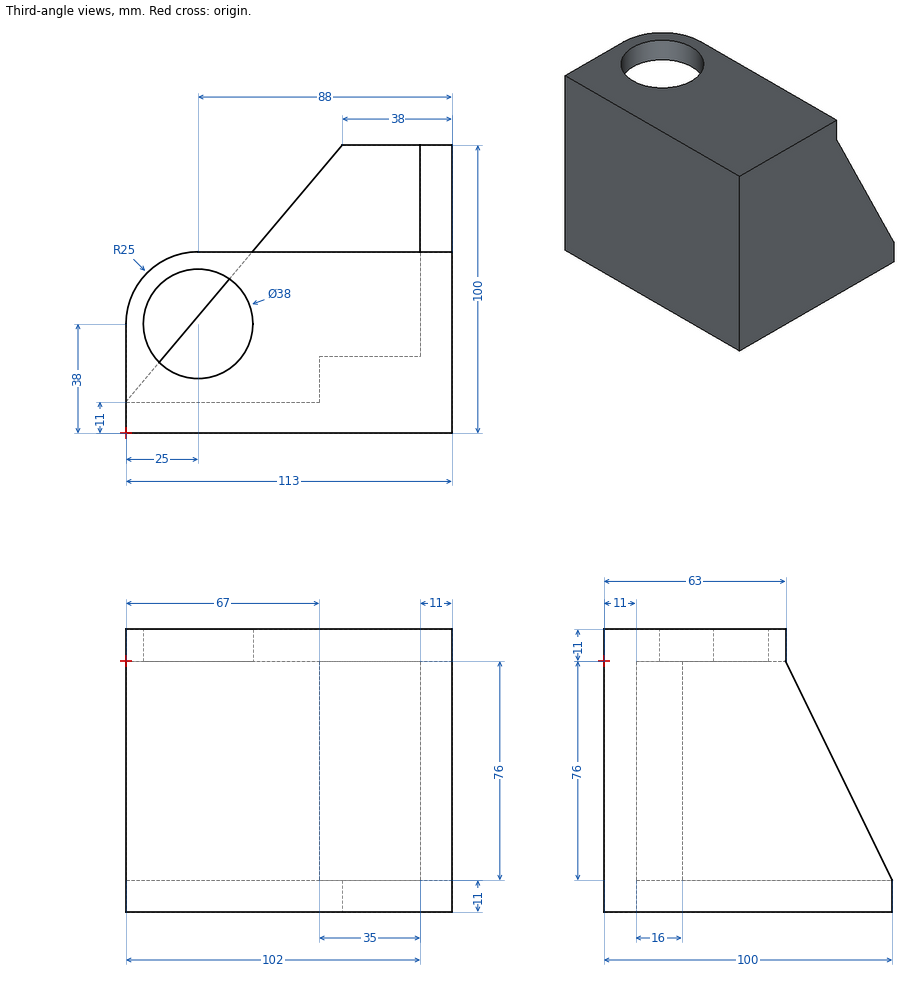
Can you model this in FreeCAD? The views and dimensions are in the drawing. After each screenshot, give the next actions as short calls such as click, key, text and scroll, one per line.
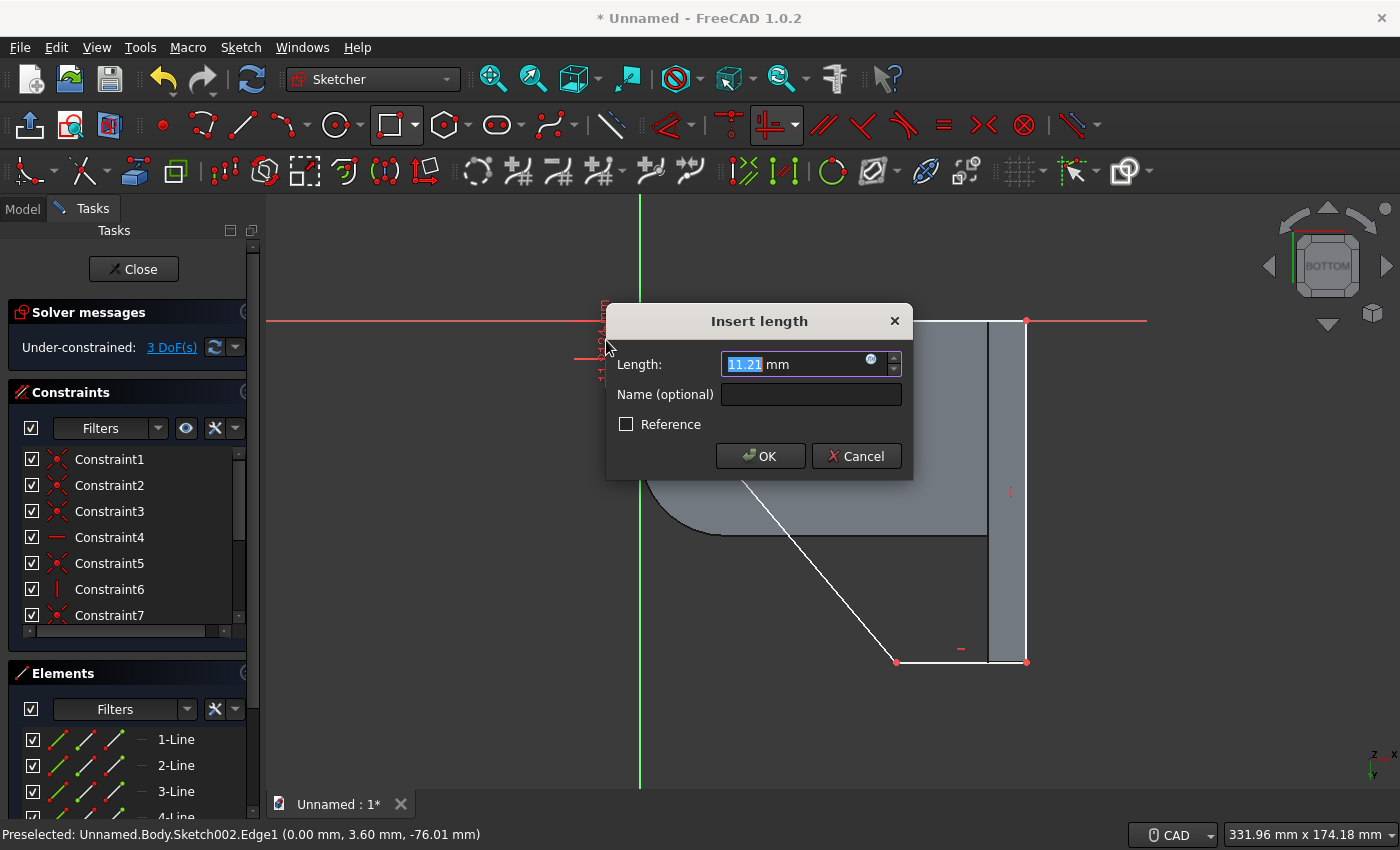
text(11)
key(Return)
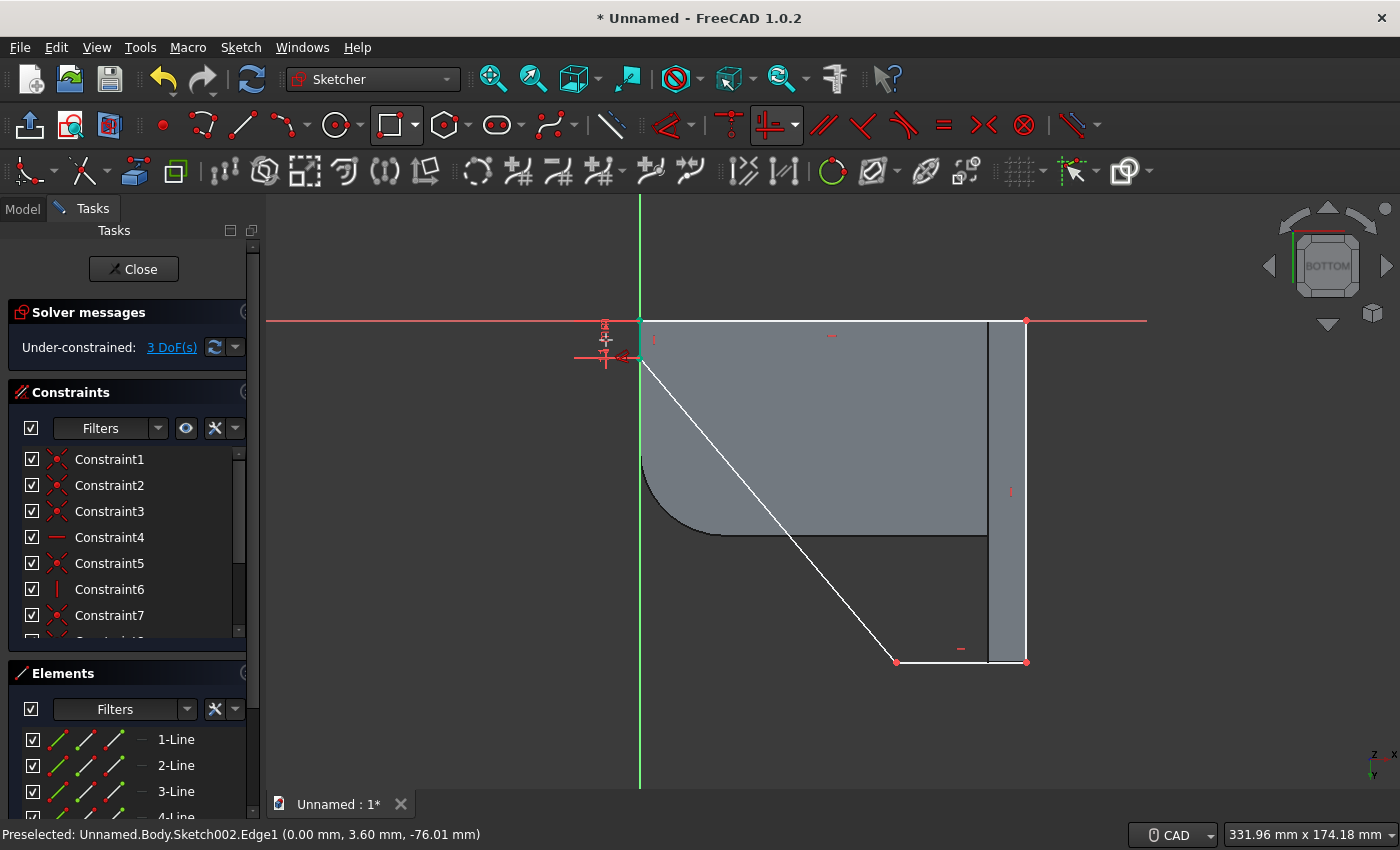
click(935, 663)
click(961, 697)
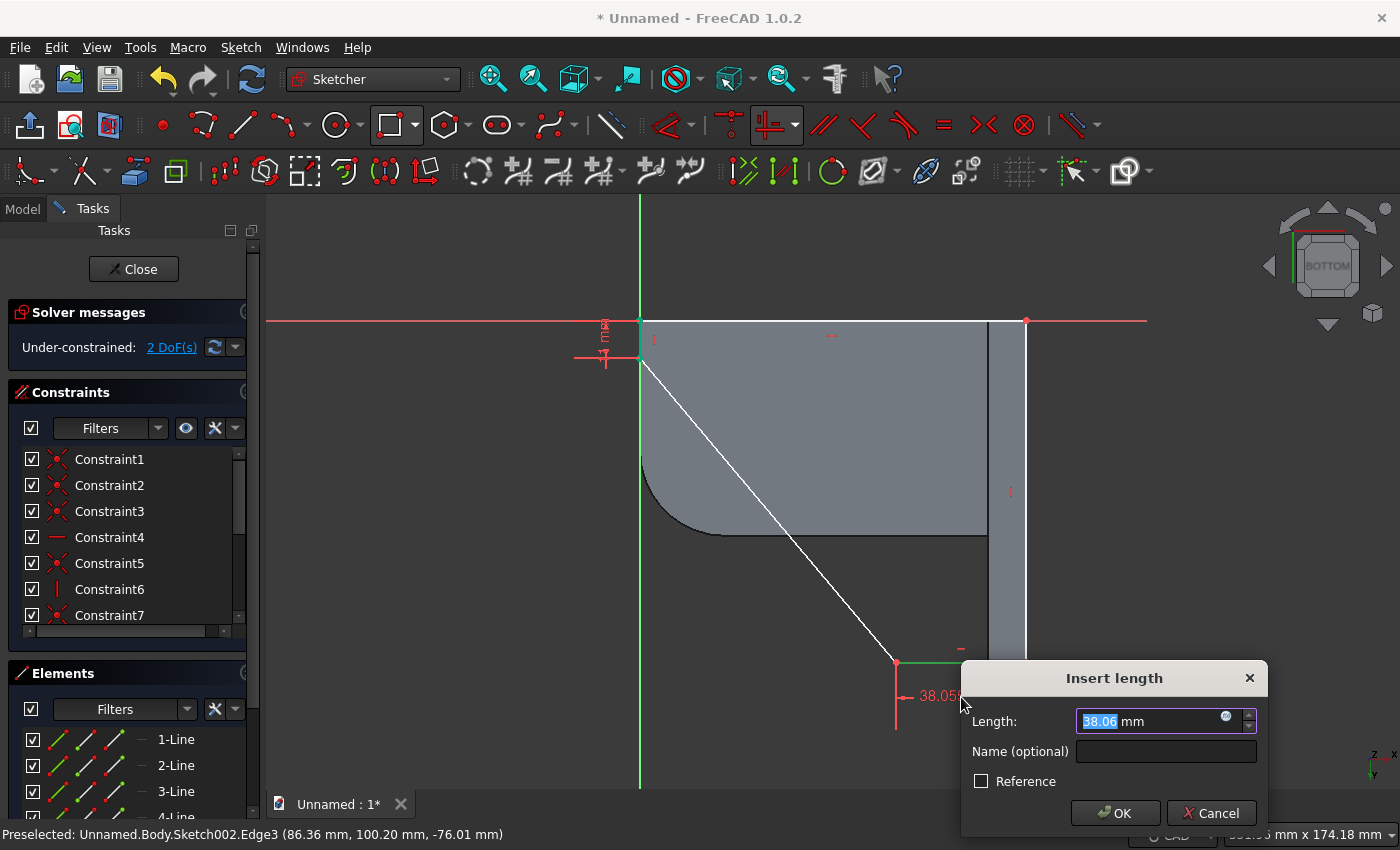
text(38)
key(Return)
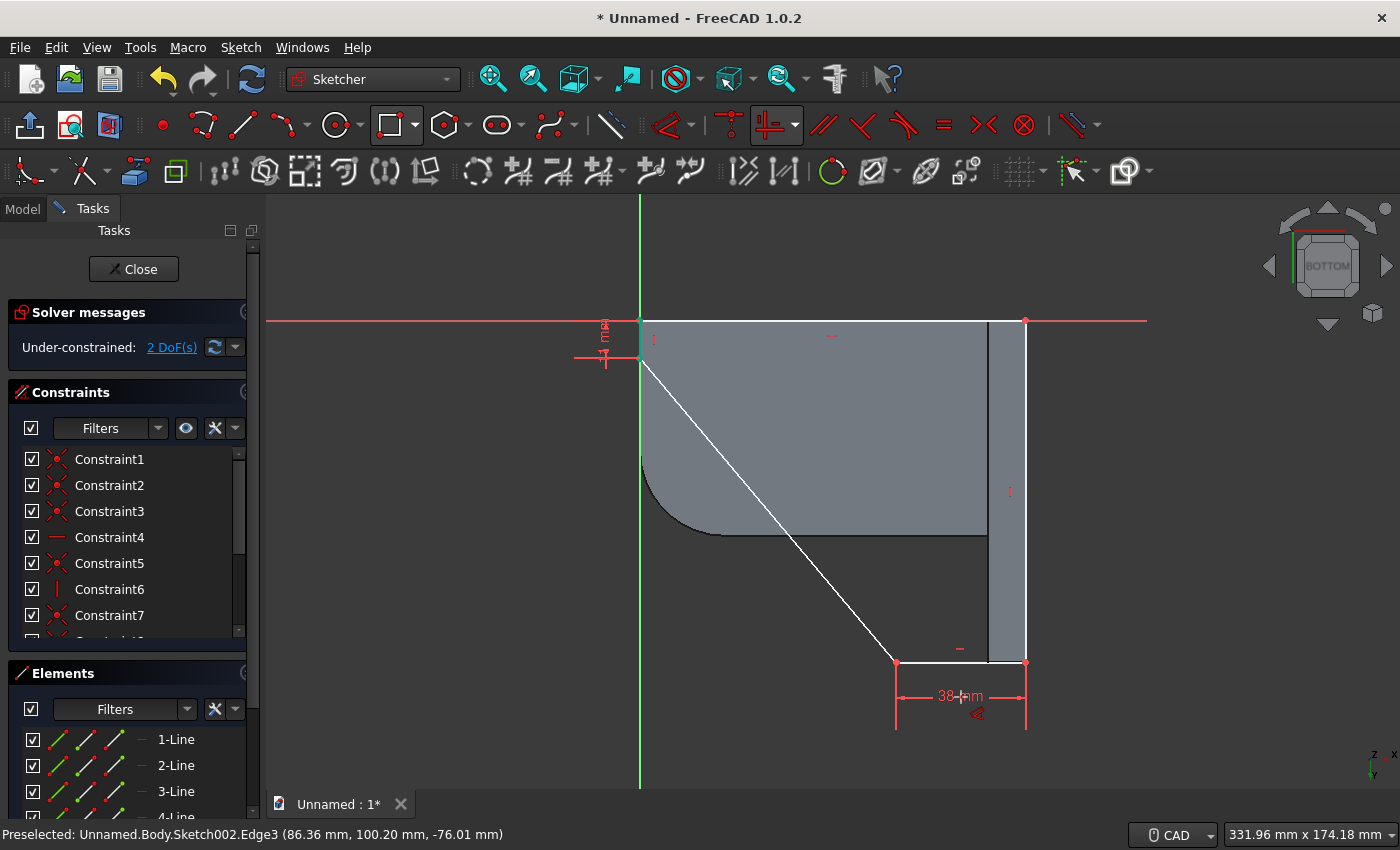
click(1026, 560)
click(1060, 492)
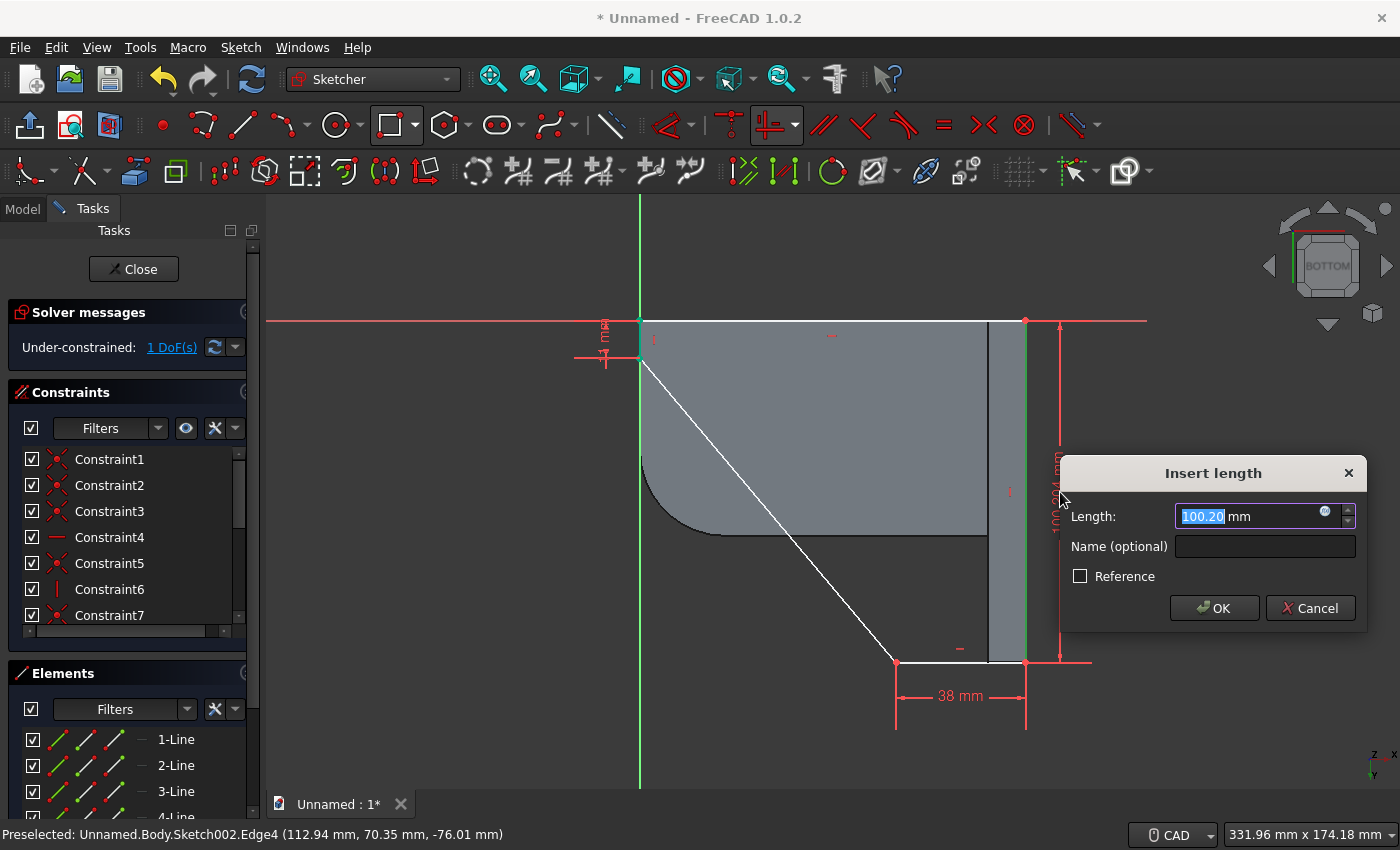
text(100)
key(Return)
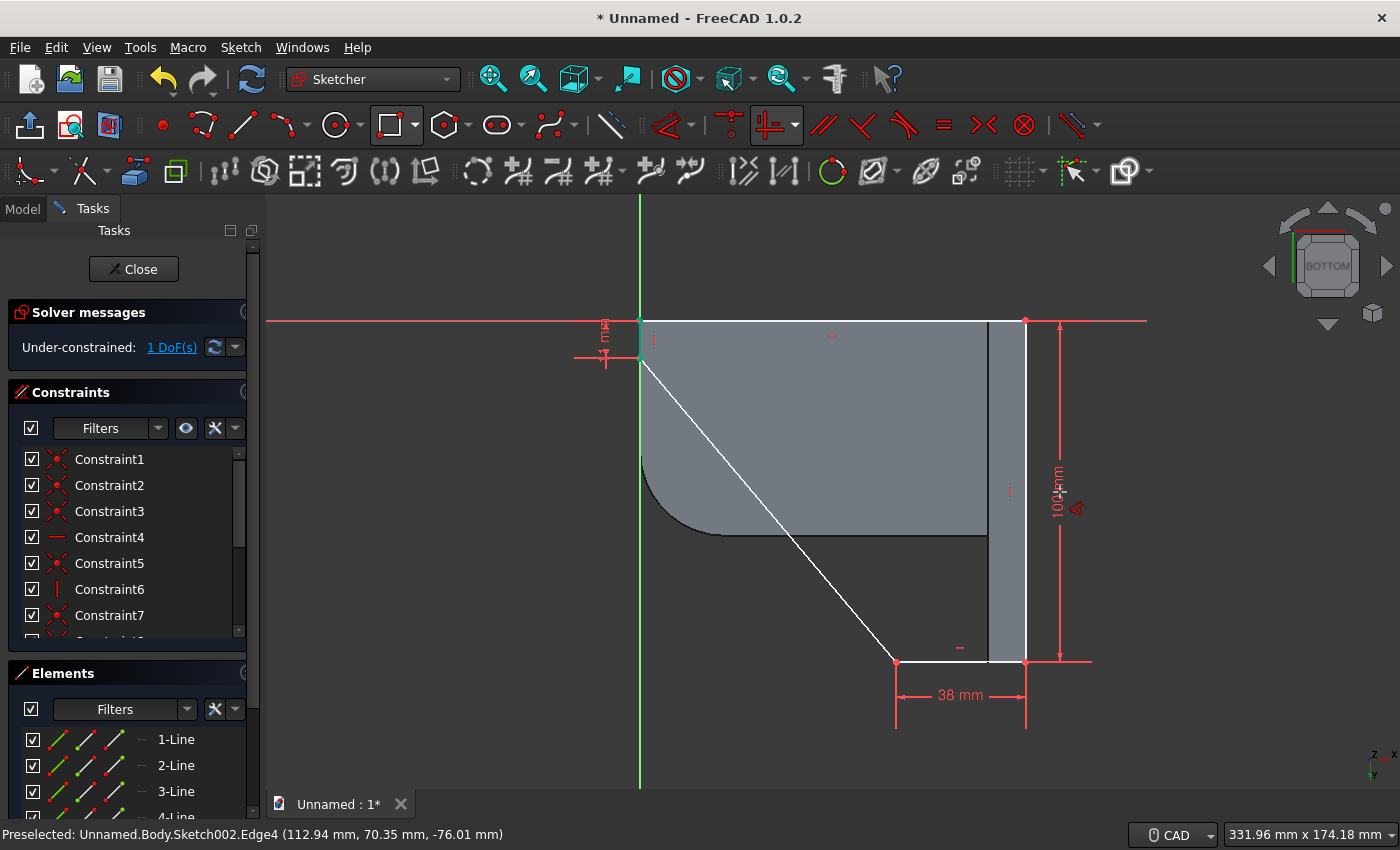
click(910, 321)
click(833, 287)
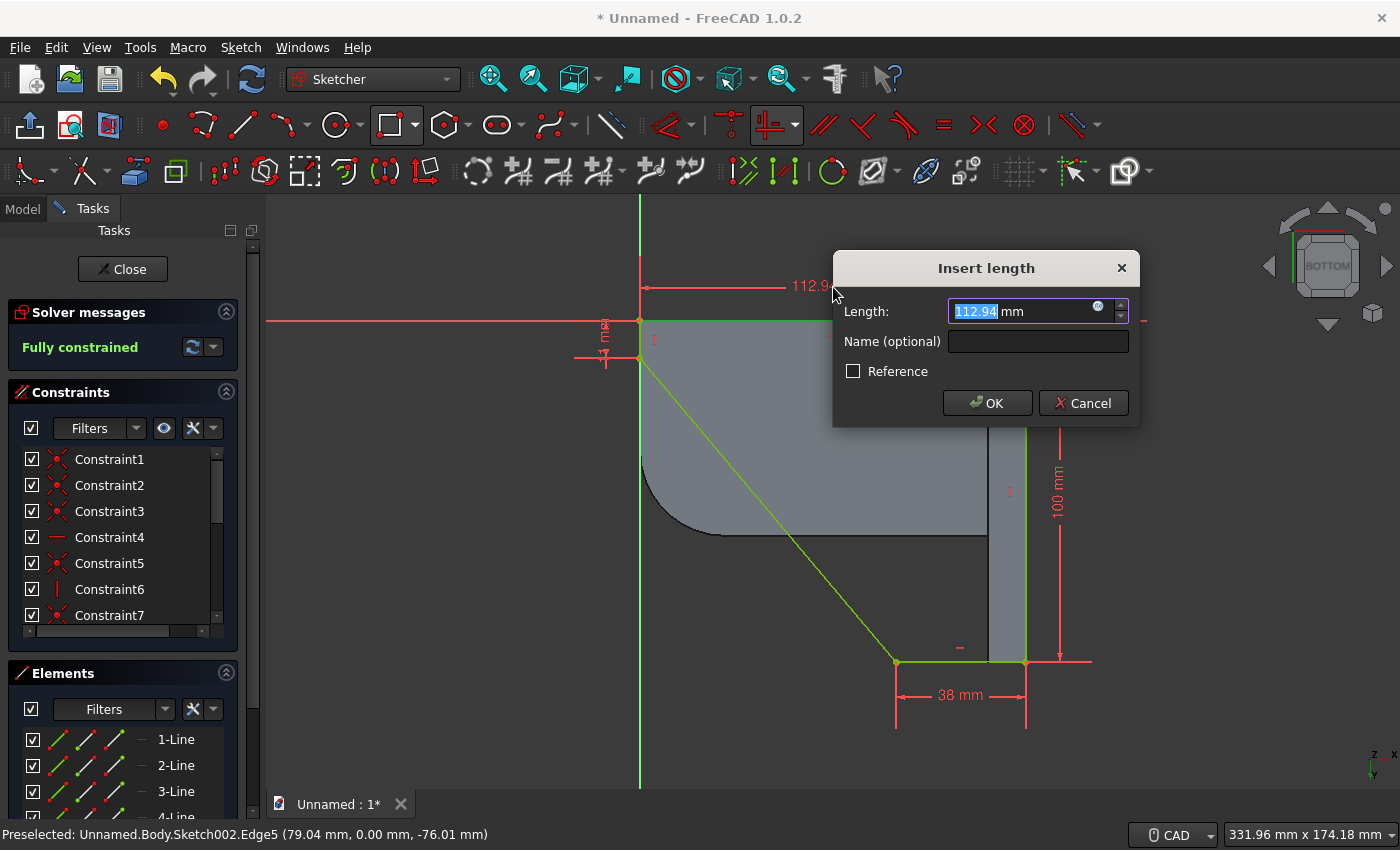
text(113)
key(Return)
key(Escape)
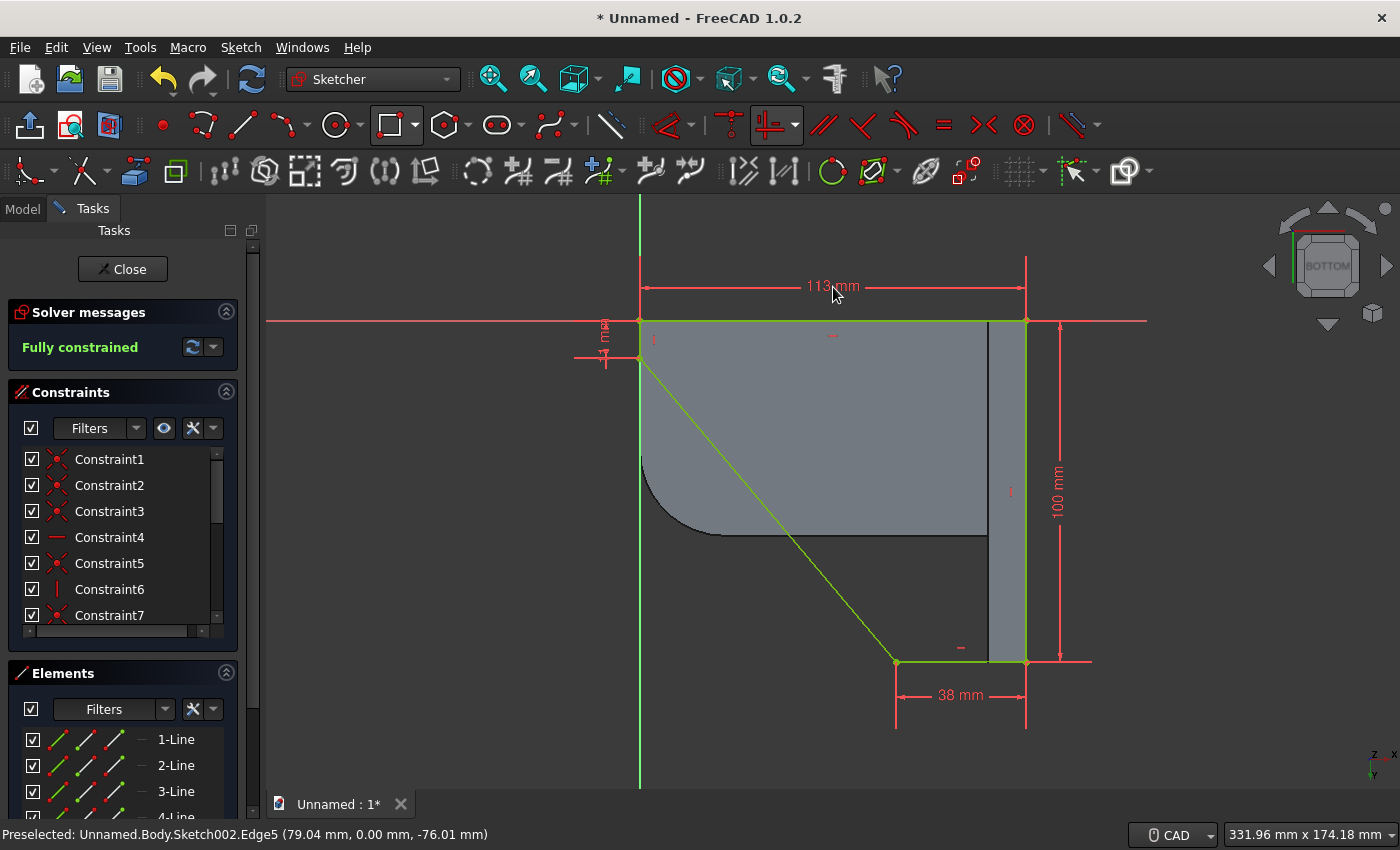
click(123, 269)